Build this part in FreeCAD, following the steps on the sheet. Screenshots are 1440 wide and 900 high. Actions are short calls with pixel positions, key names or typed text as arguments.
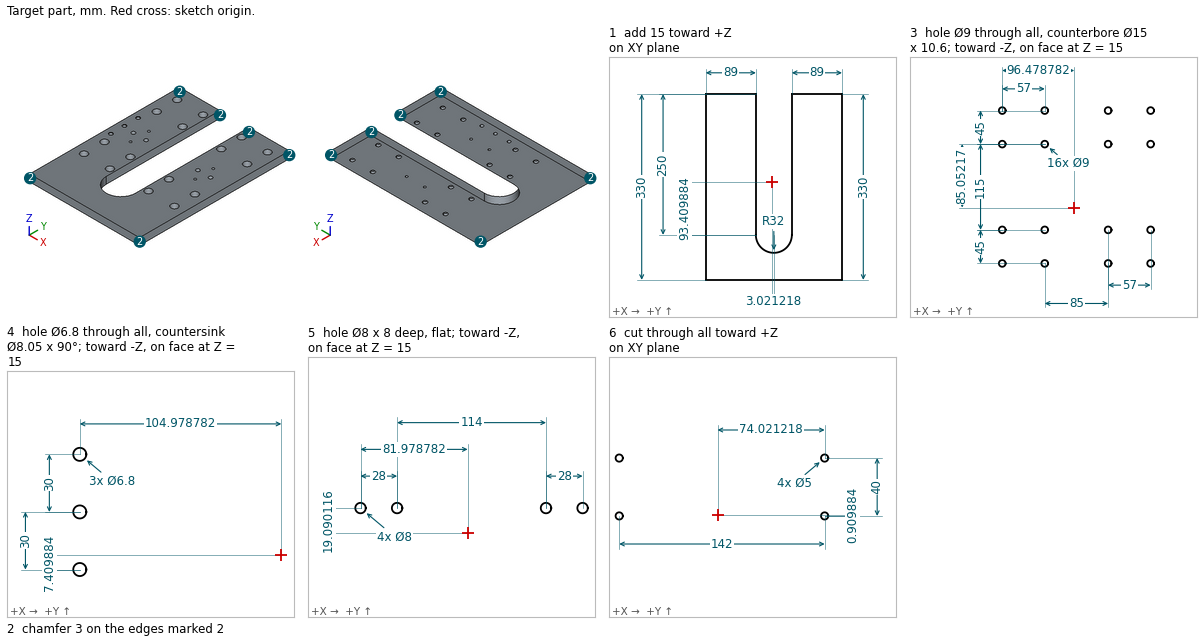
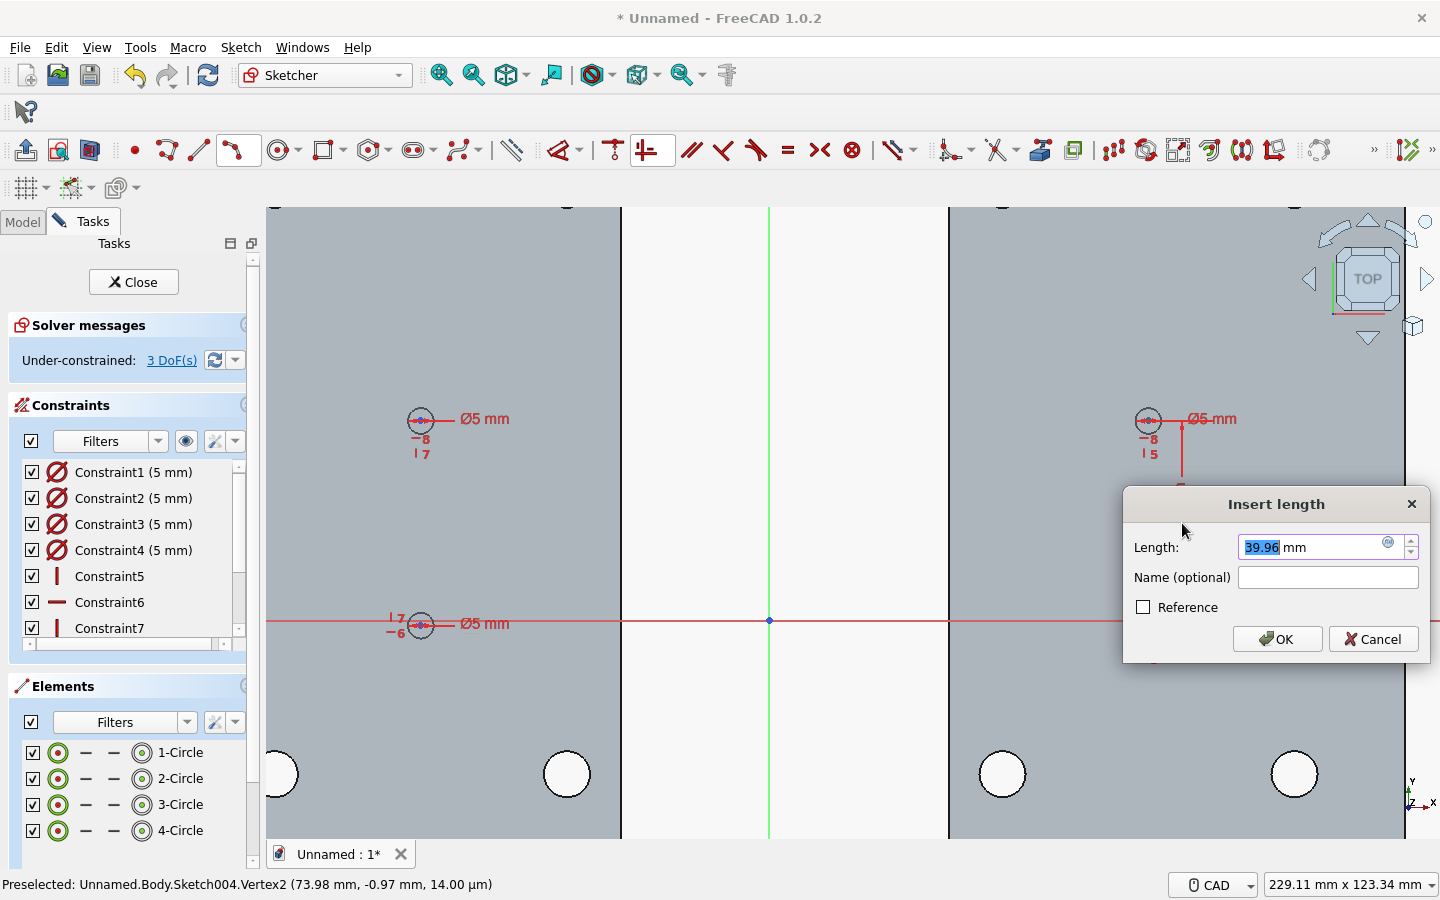
text(40)
key(Return)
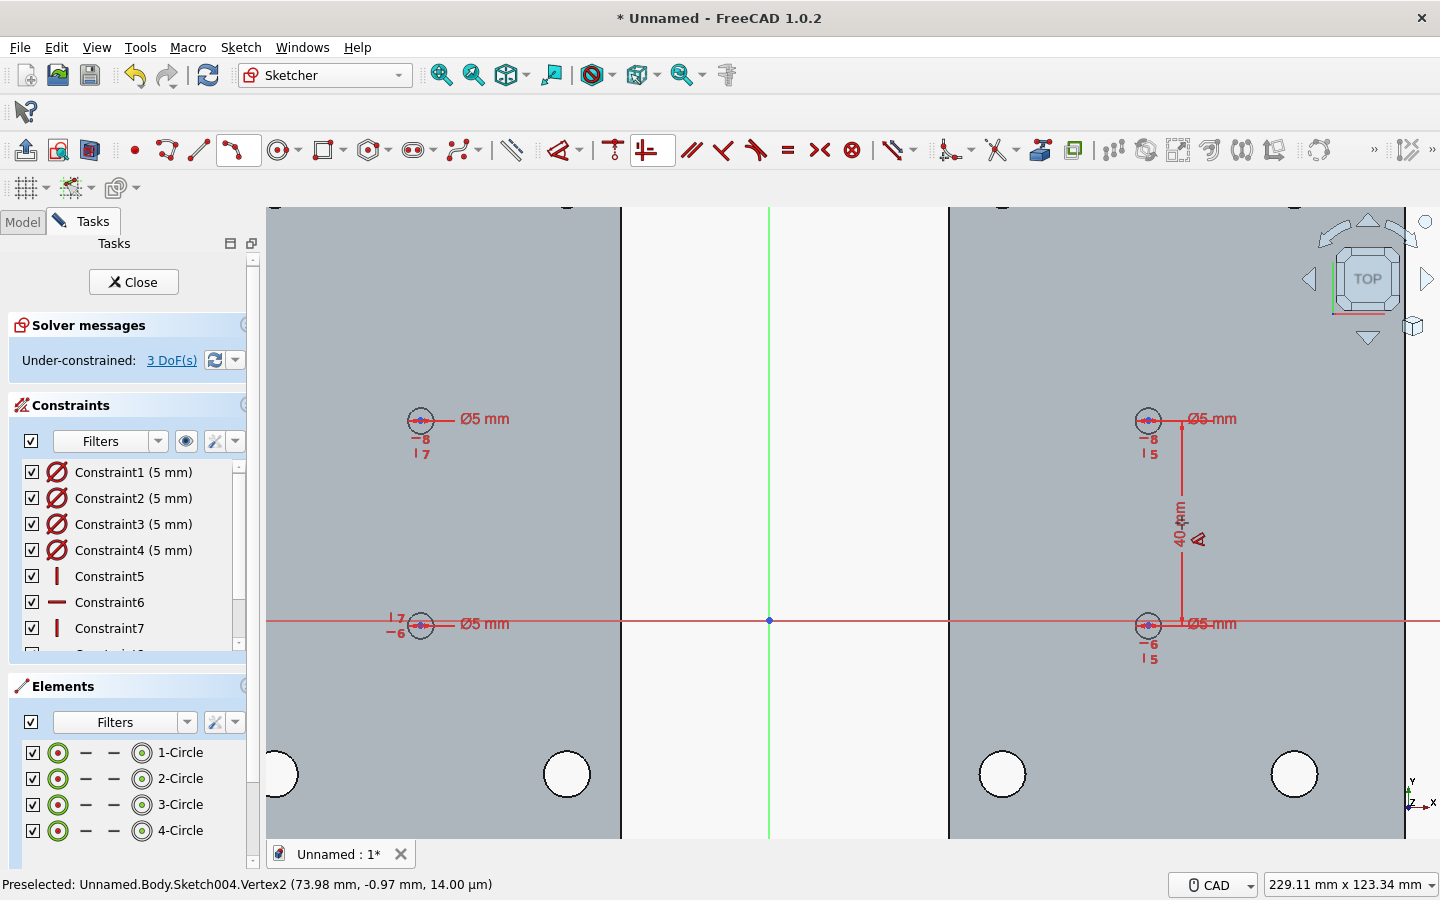
click(1148, 626)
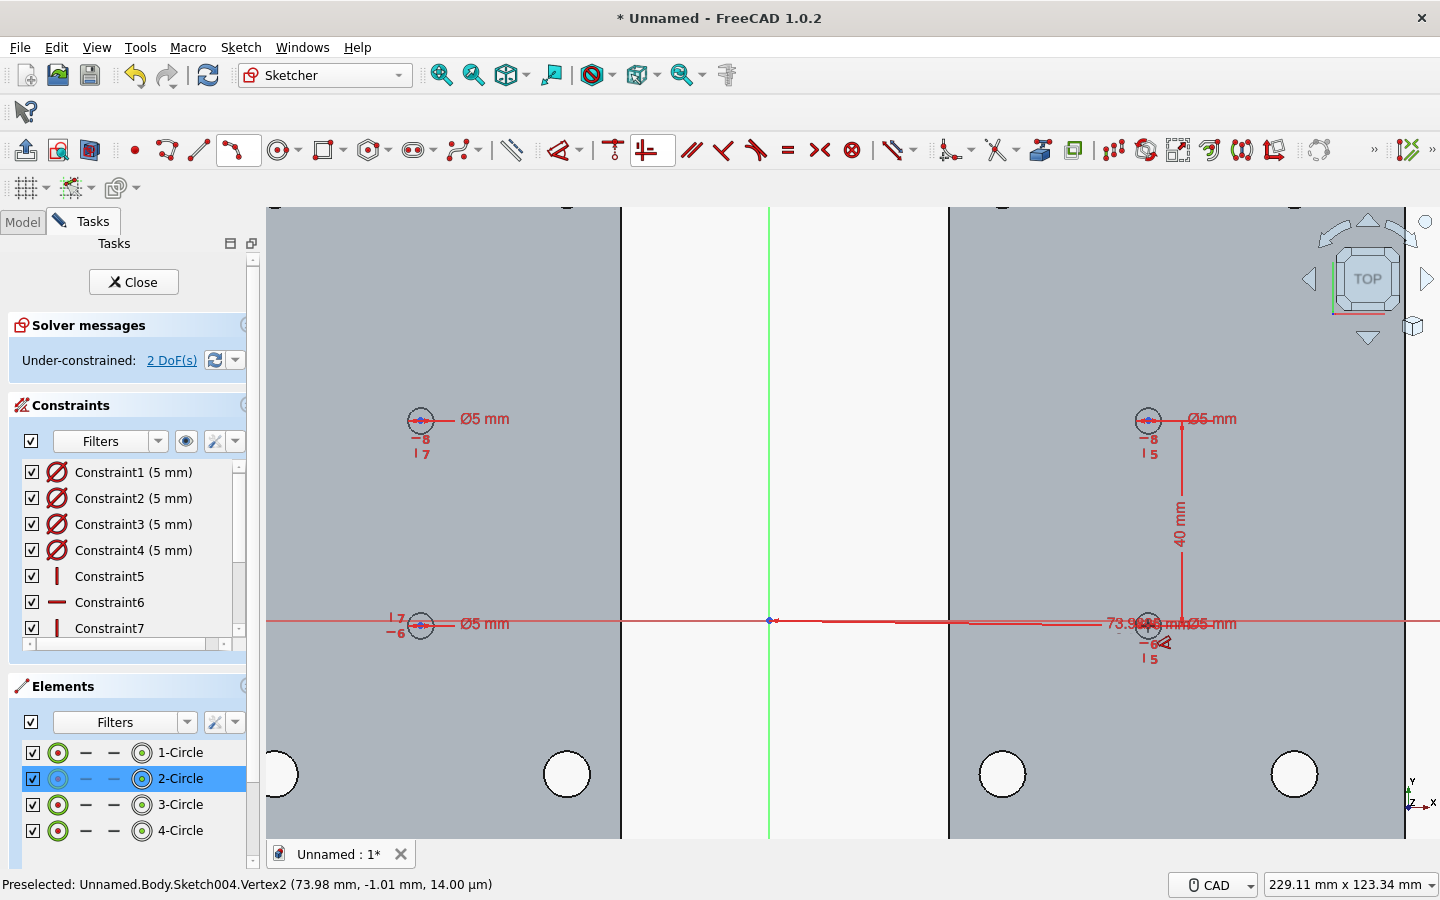
click(421, 626)
click(785, 660)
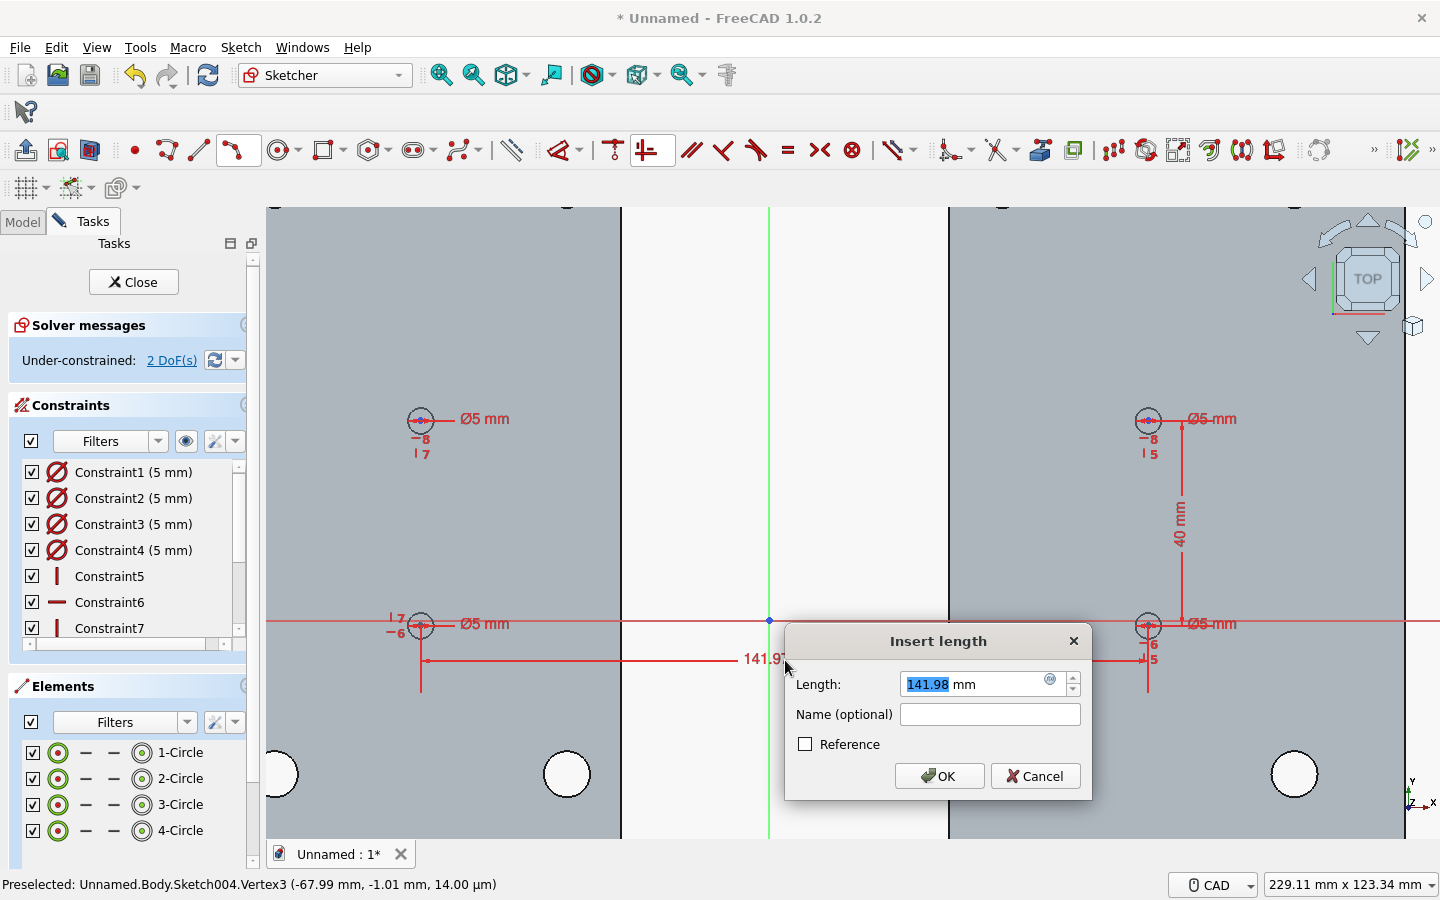
text(142)
key(Return)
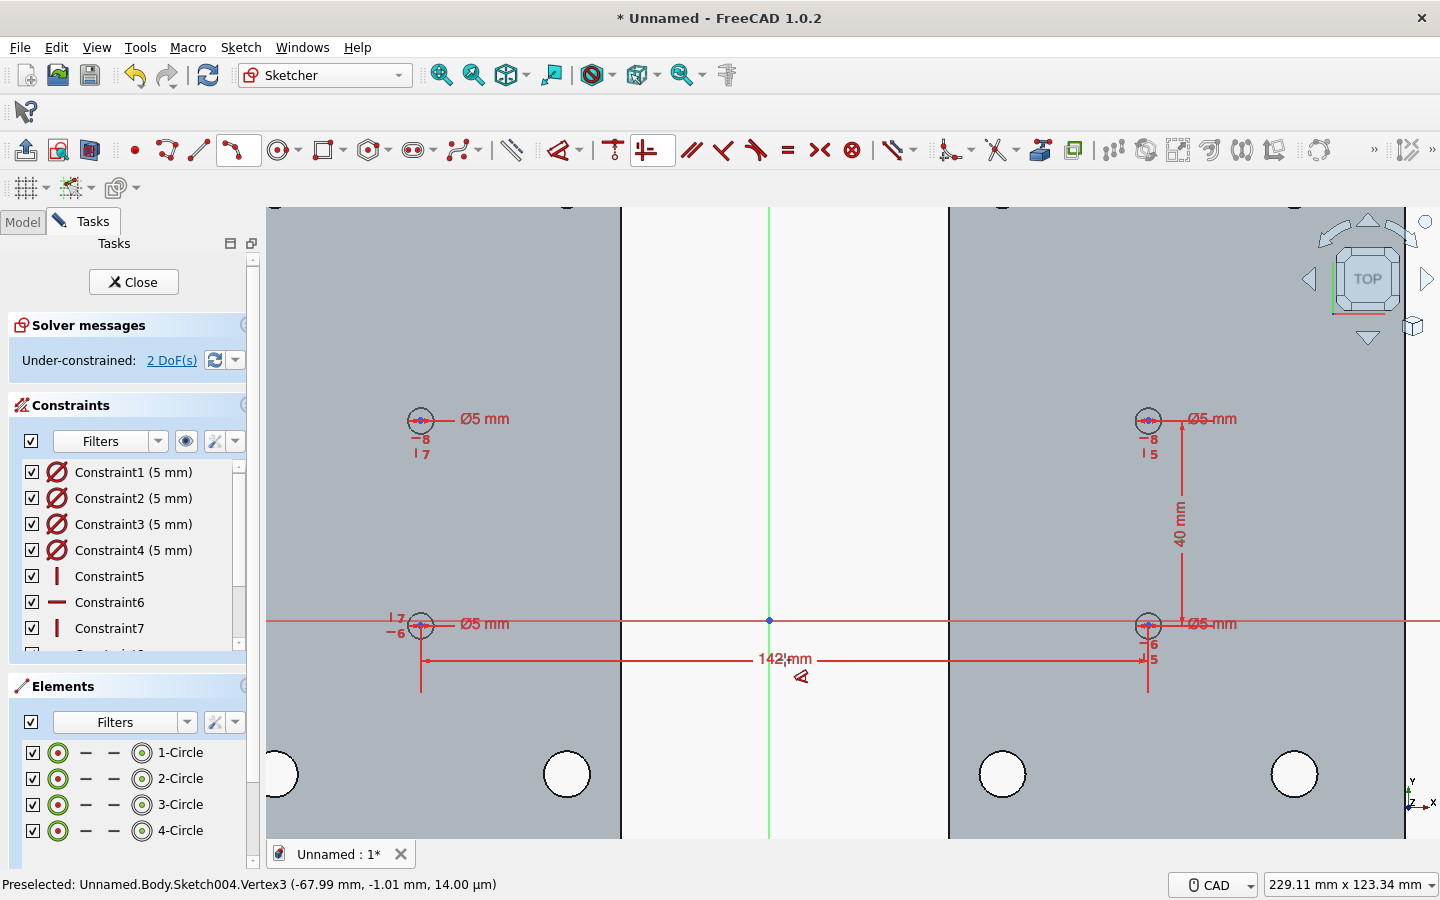
scroll(1148, 626, up, 11)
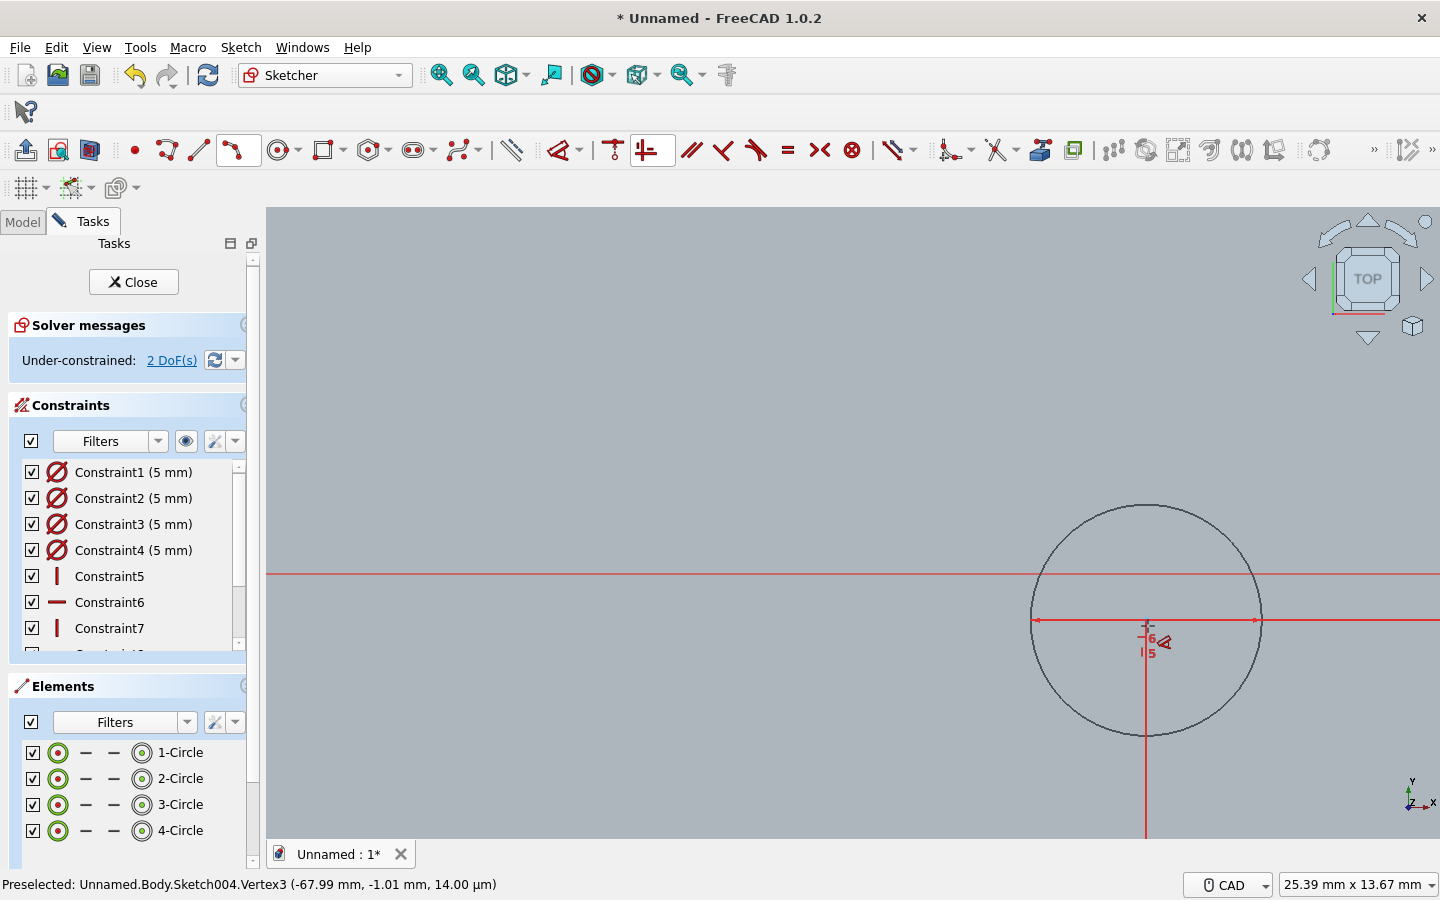
click(1146, 620)
click(1180, 597)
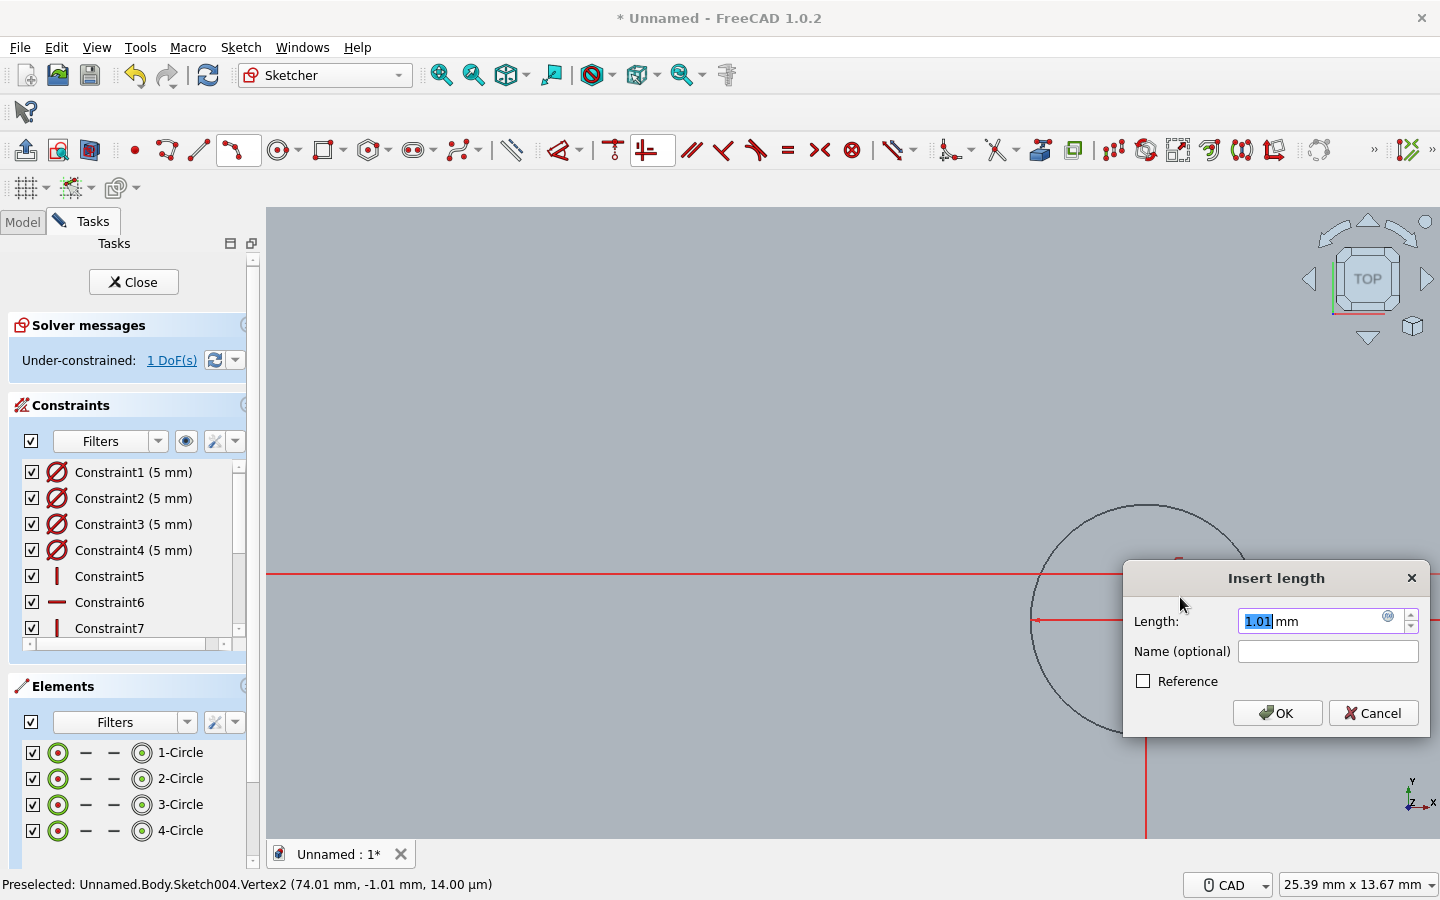
text(0.909884)
key(Return)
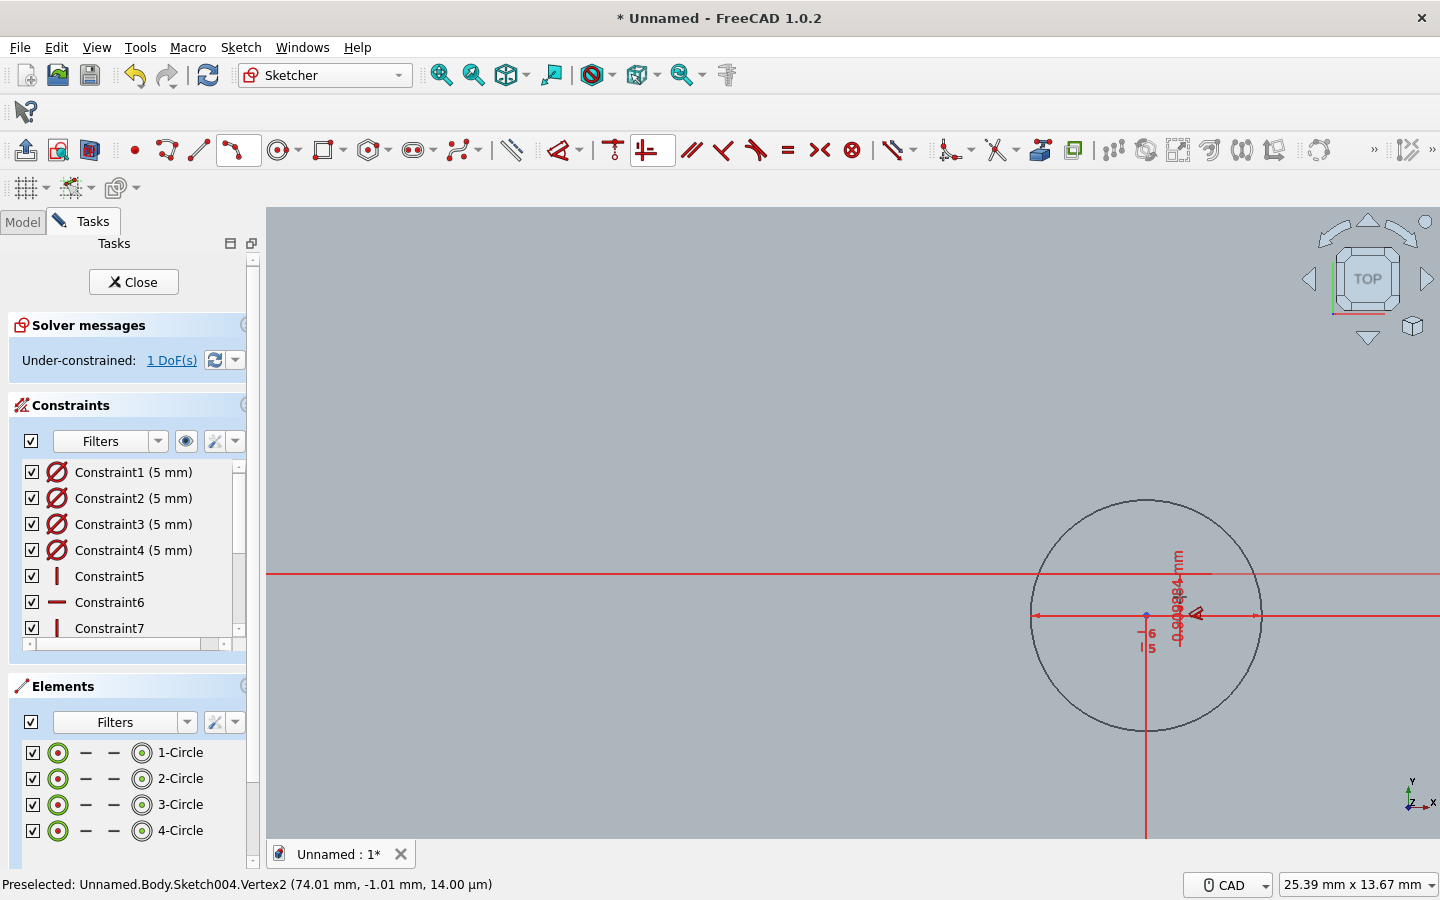
scroll(1148, 627, down, 11)